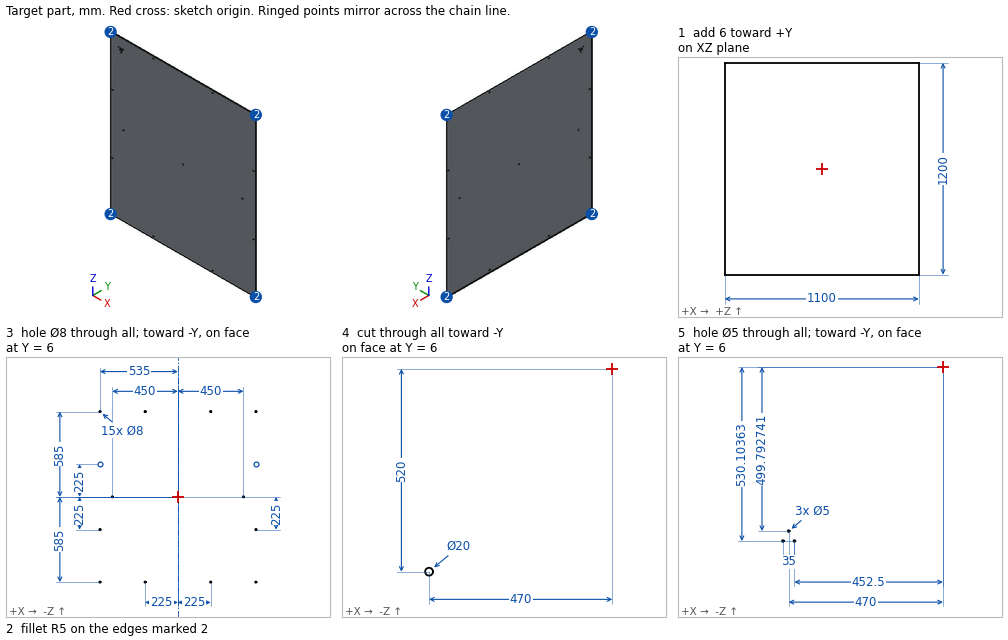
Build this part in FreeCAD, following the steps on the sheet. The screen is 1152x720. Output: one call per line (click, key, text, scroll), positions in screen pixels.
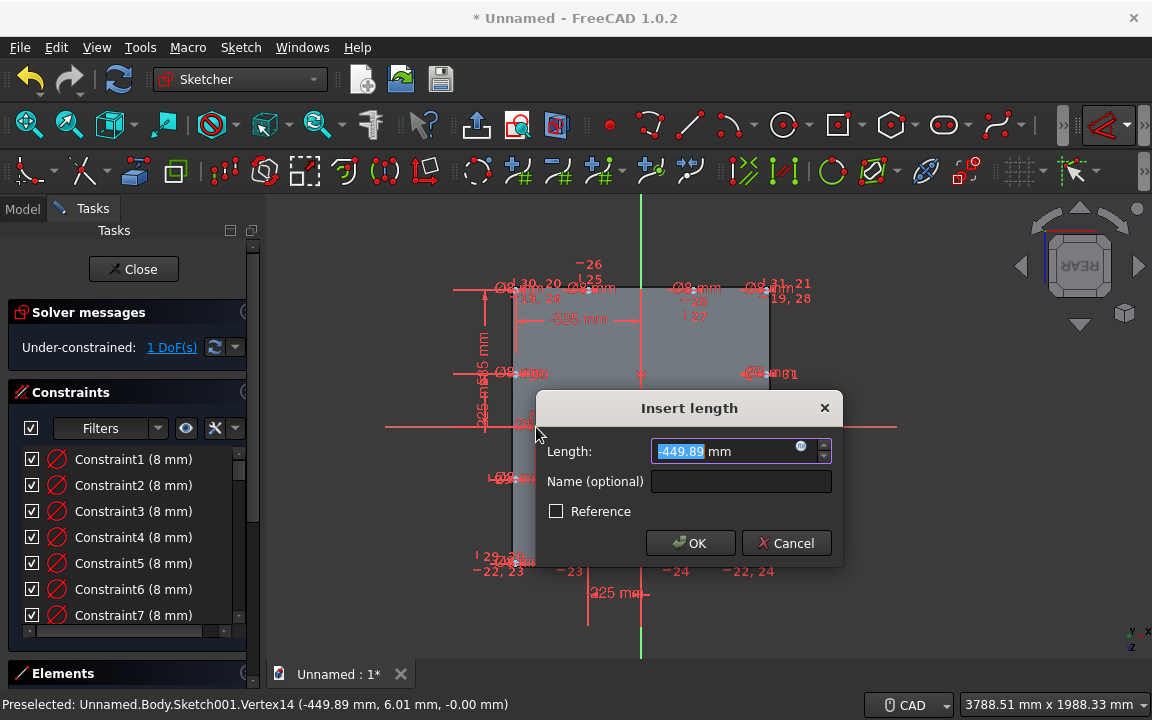
text(-450)
key(Return)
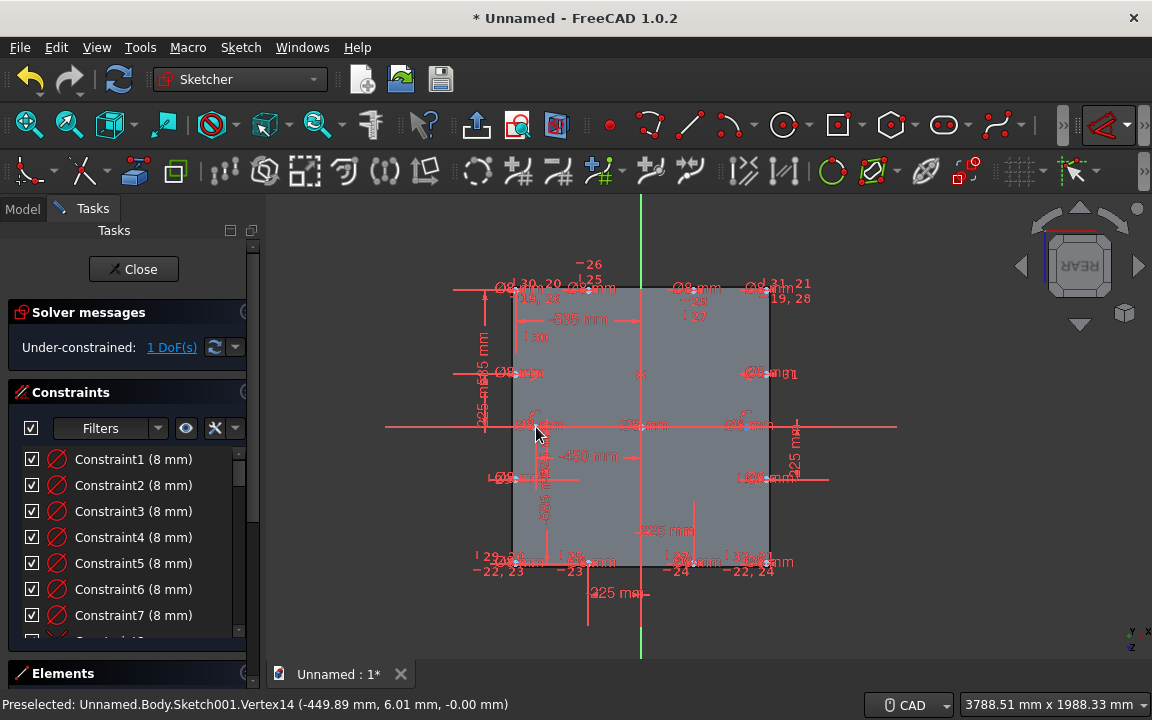
click(746, 427)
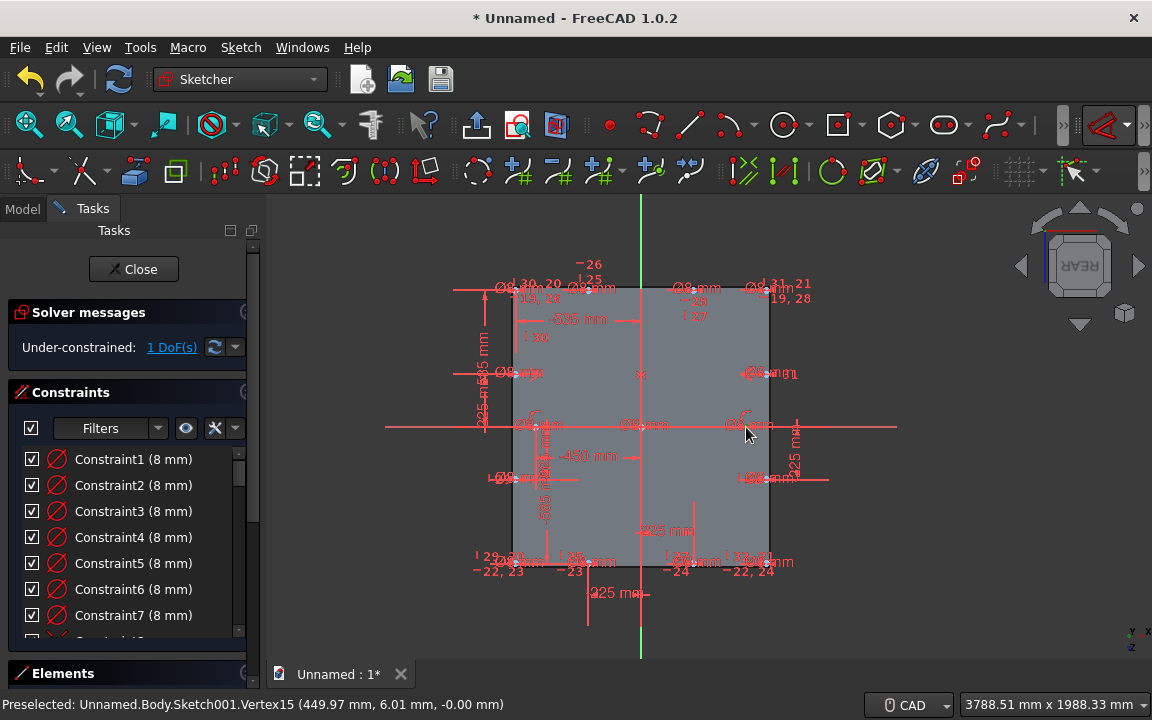
click(1130, 126)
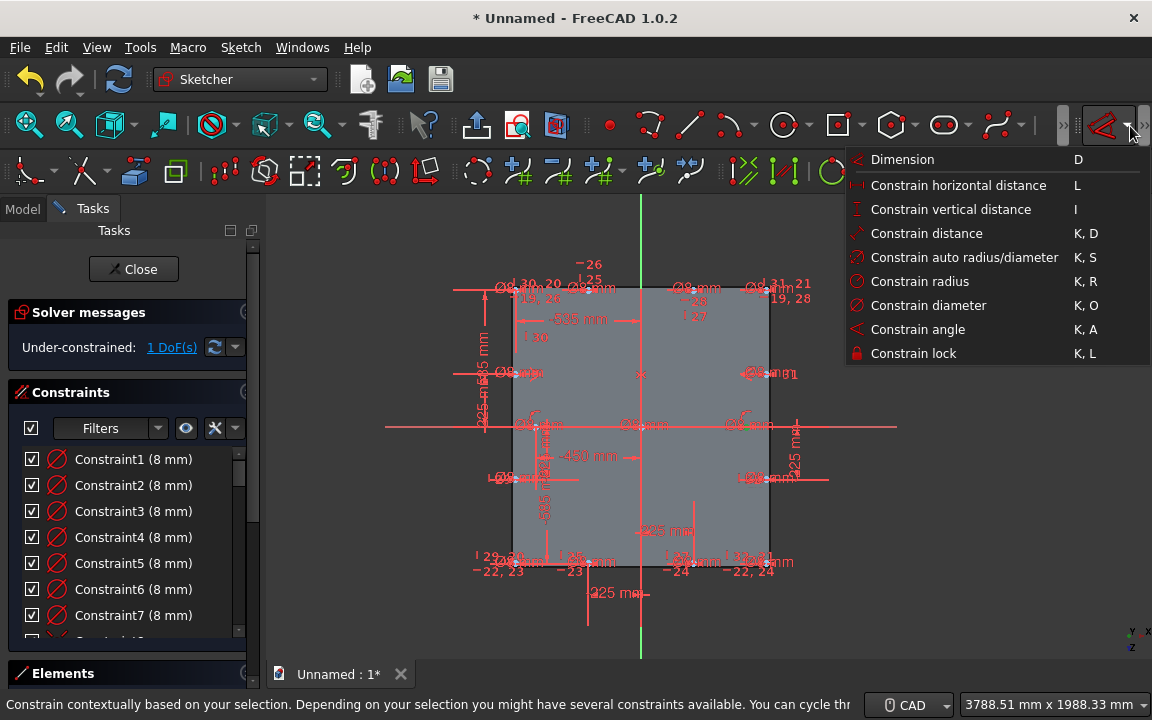
click(998, 185)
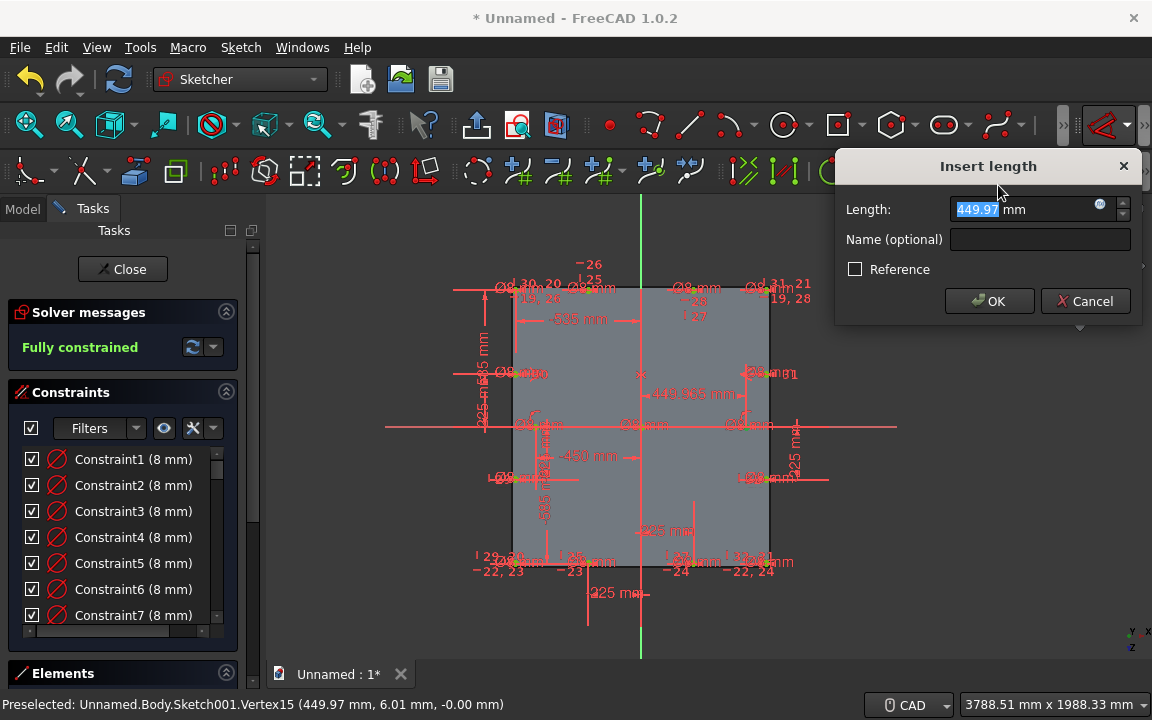
text(450)
key(Return)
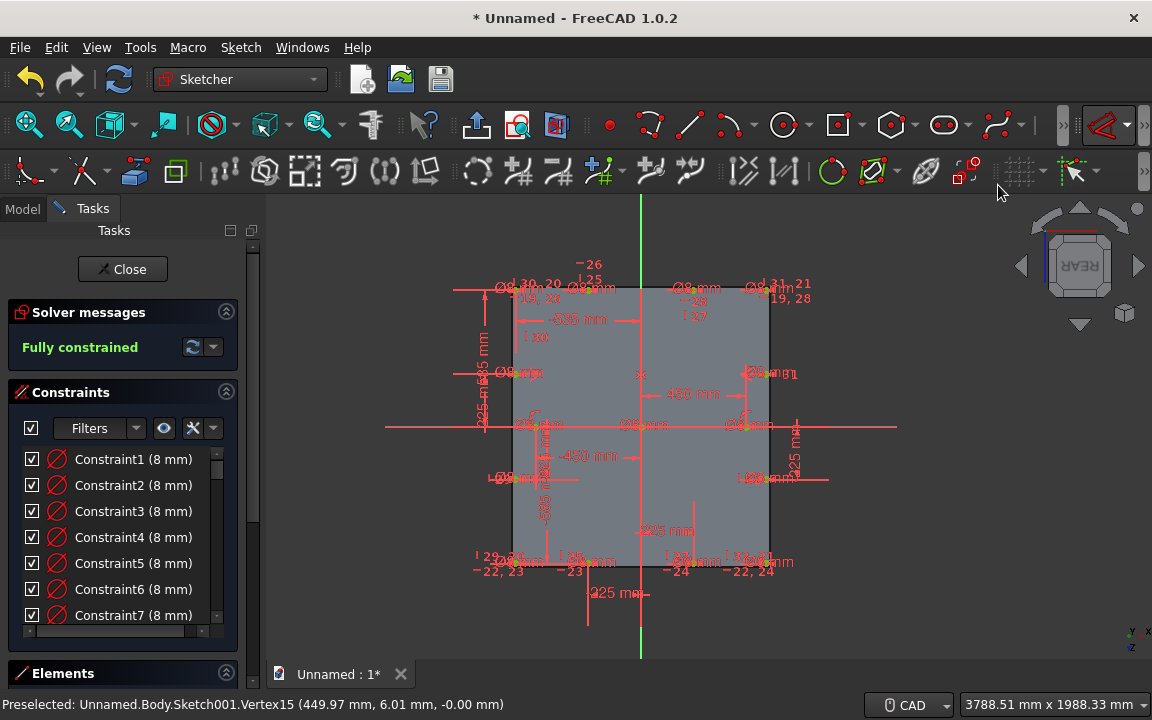
click(123, 269)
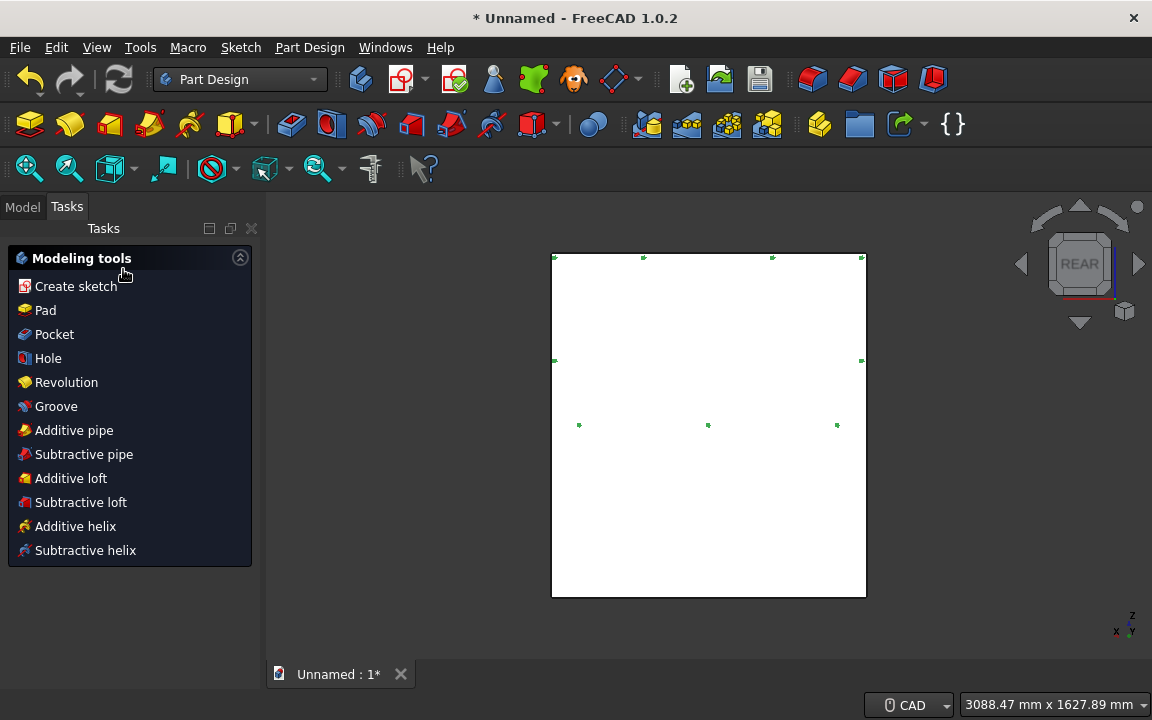
click(332, 124)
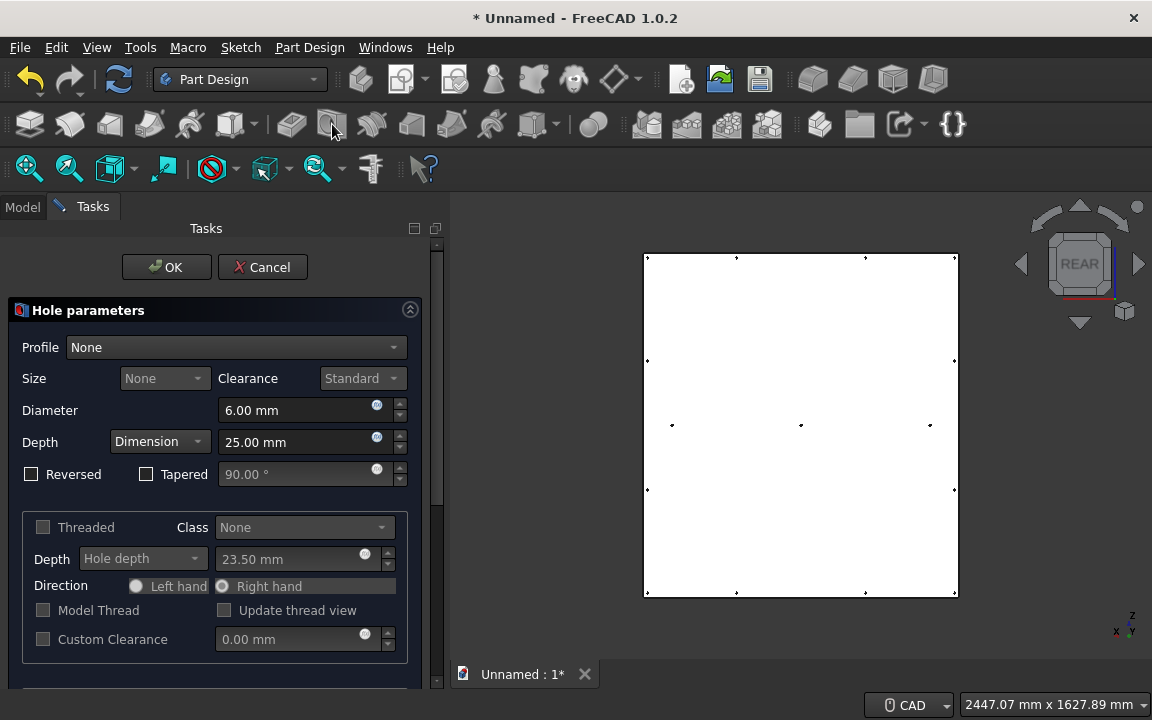
triple_click(305, 410)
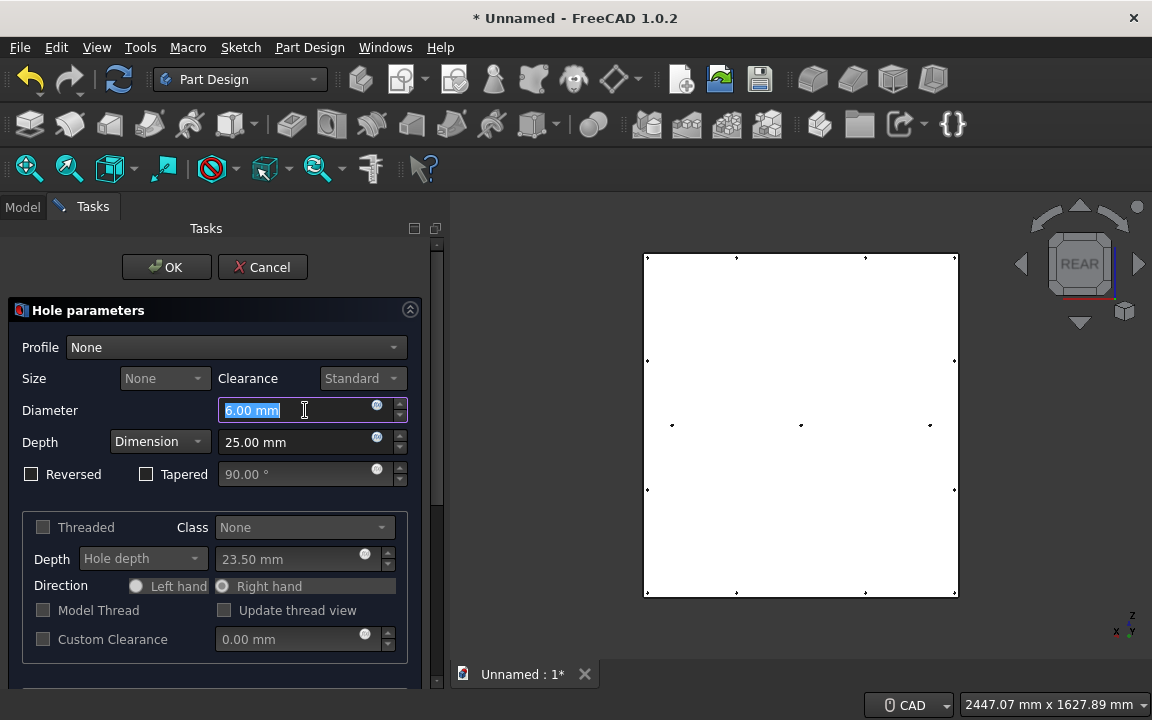
text(8)
key(Tab)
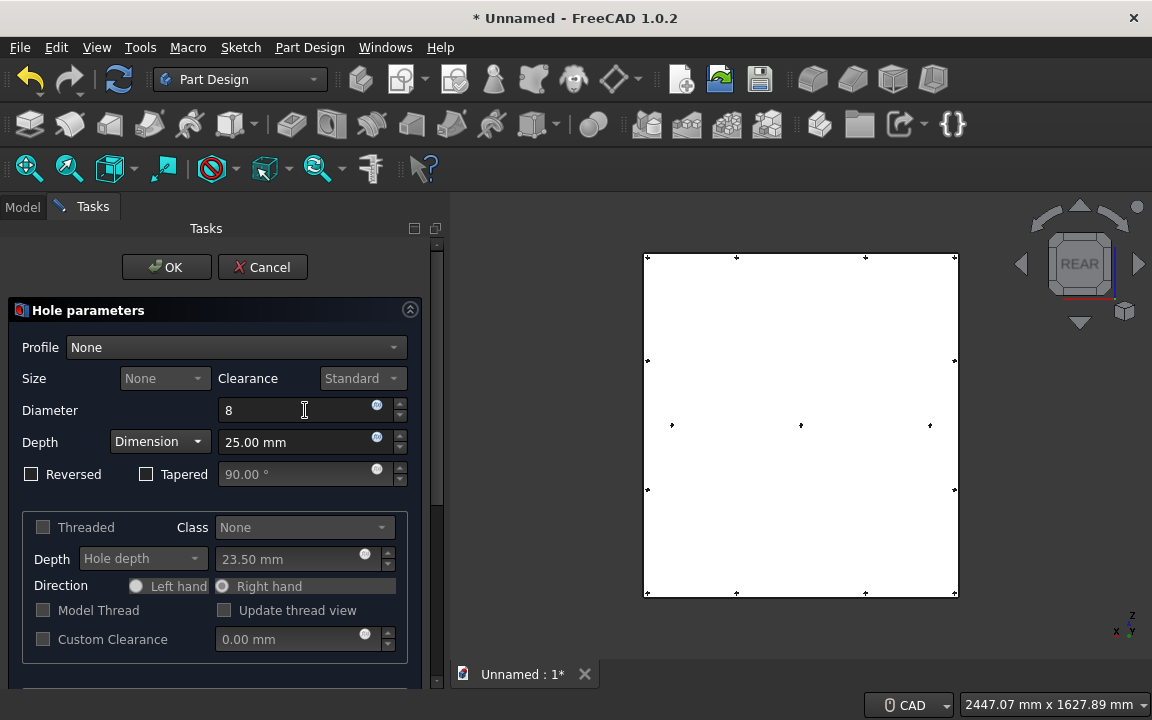
click(161, 442)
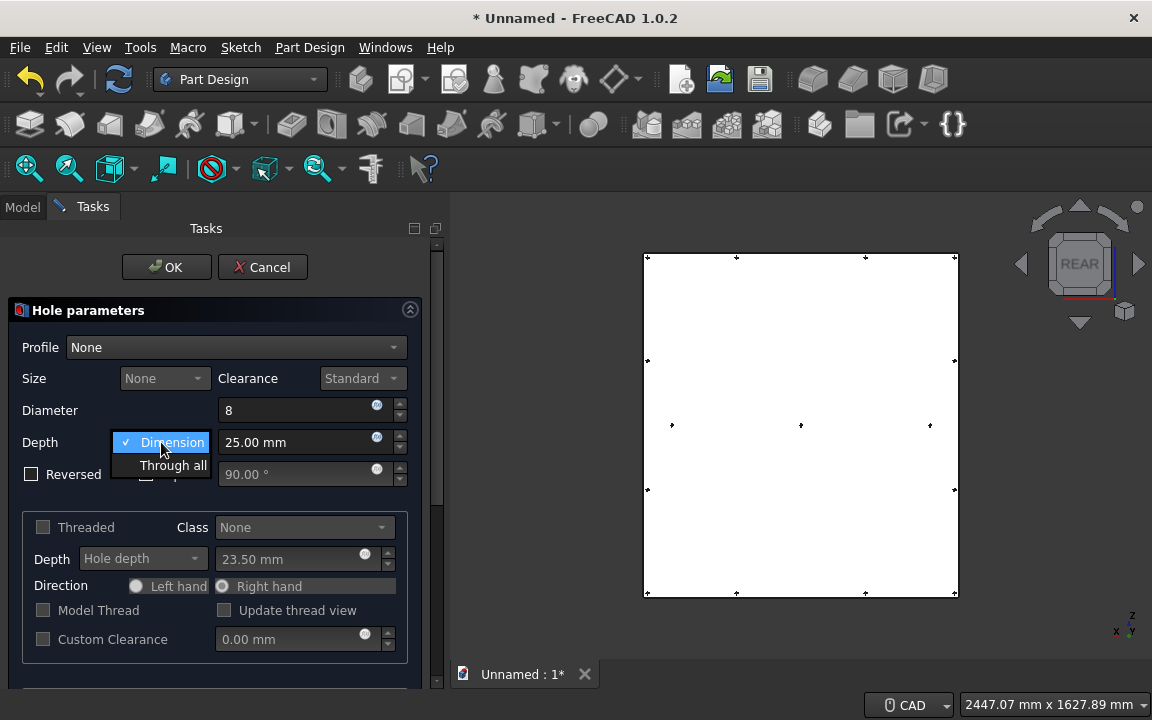
click(160, 466)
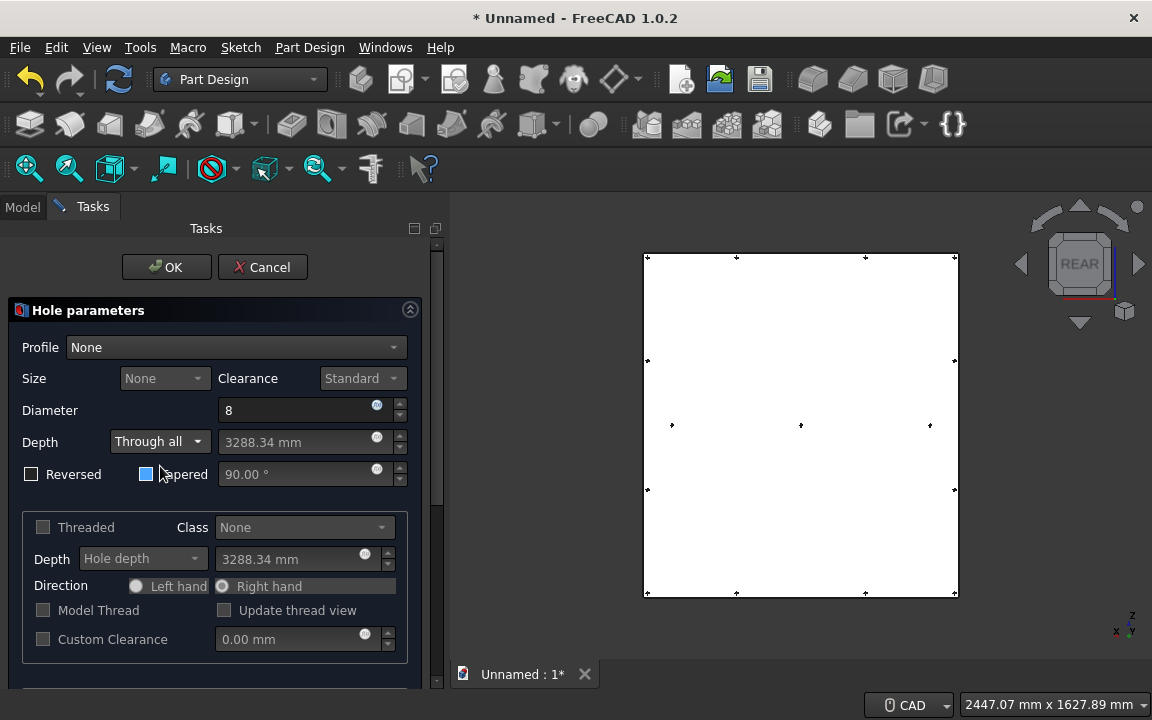
click(167, 267)